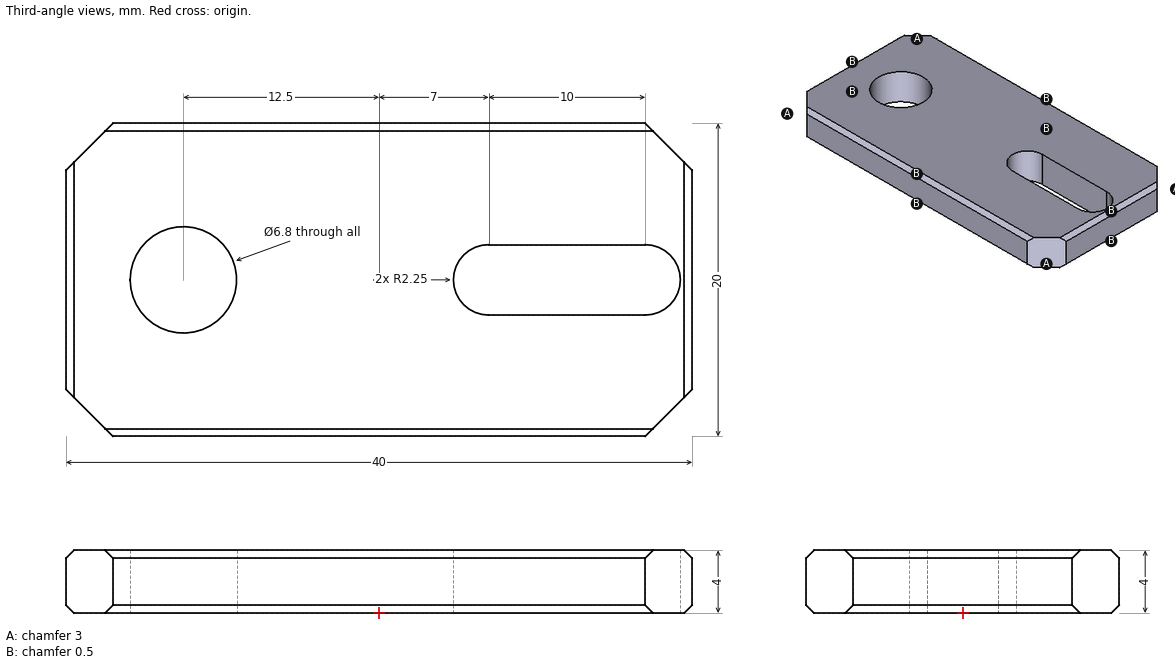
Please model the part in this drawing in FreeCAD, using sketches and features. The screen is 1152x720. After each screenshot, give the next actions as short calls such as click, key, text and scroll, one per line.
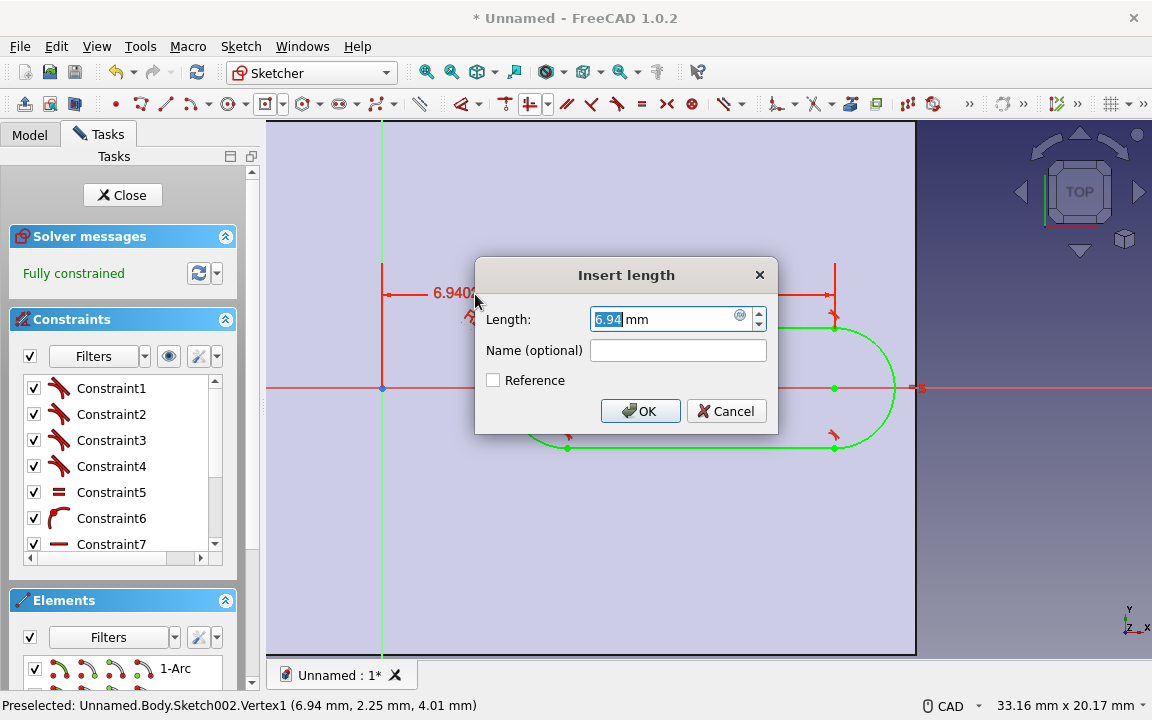
text(7)
key(Return)
key(Escape)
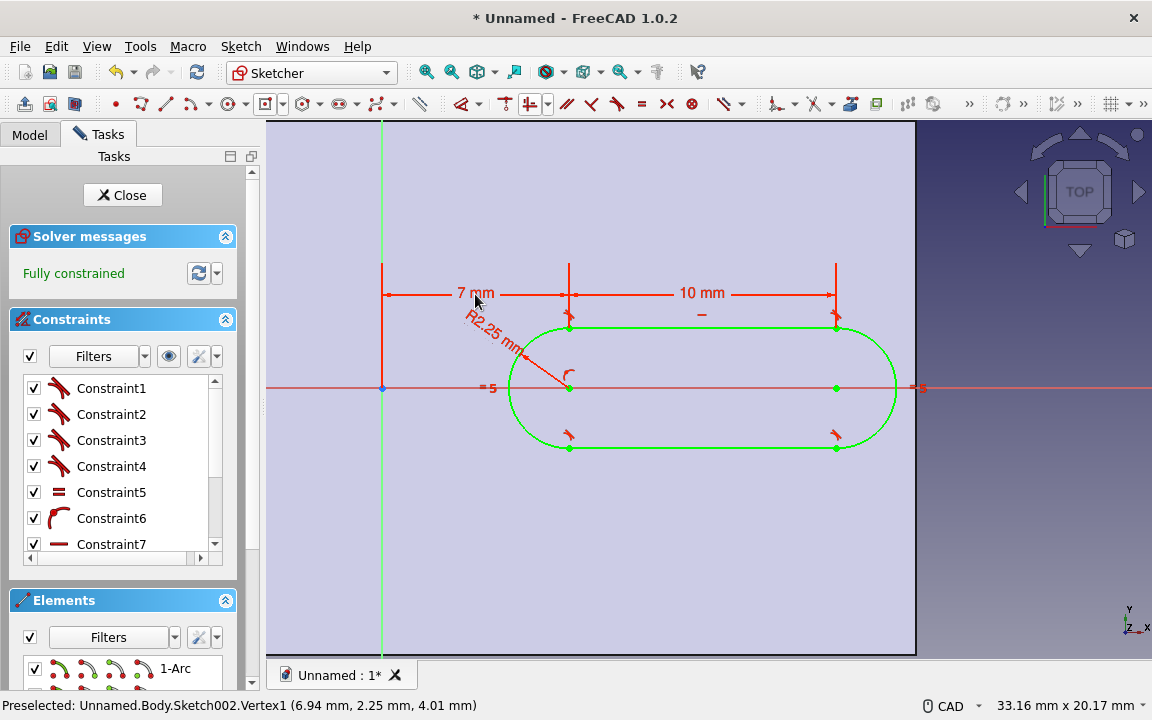
click(123, 195)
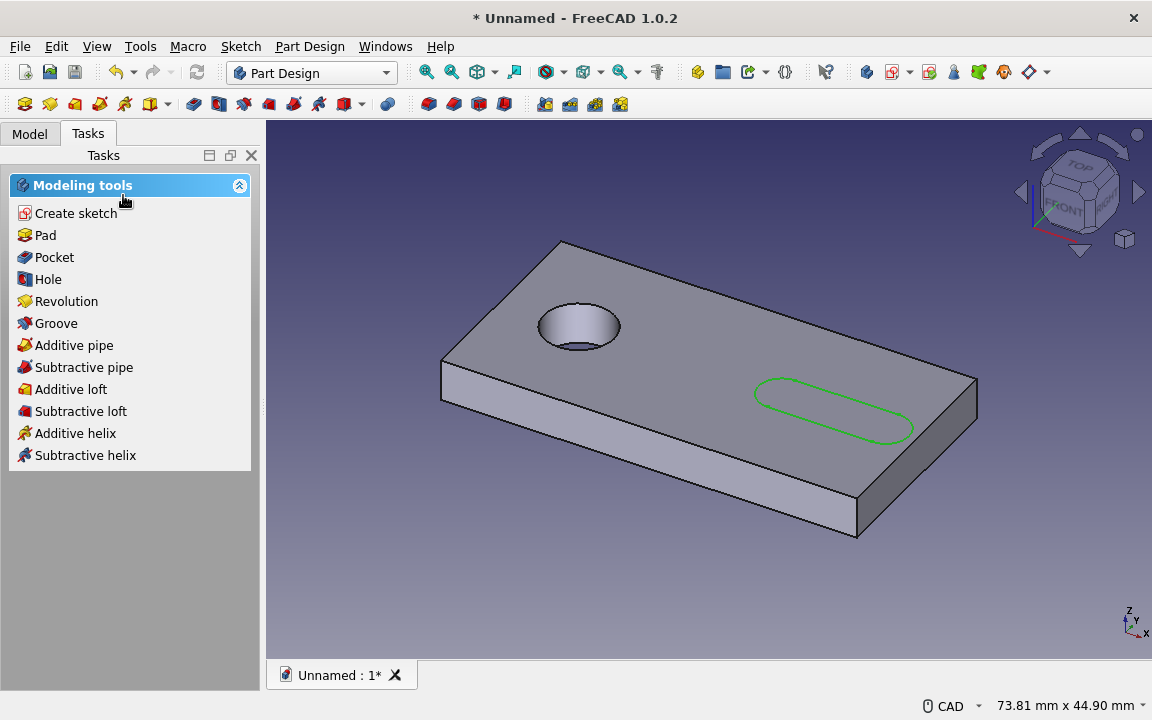
click(194, 104)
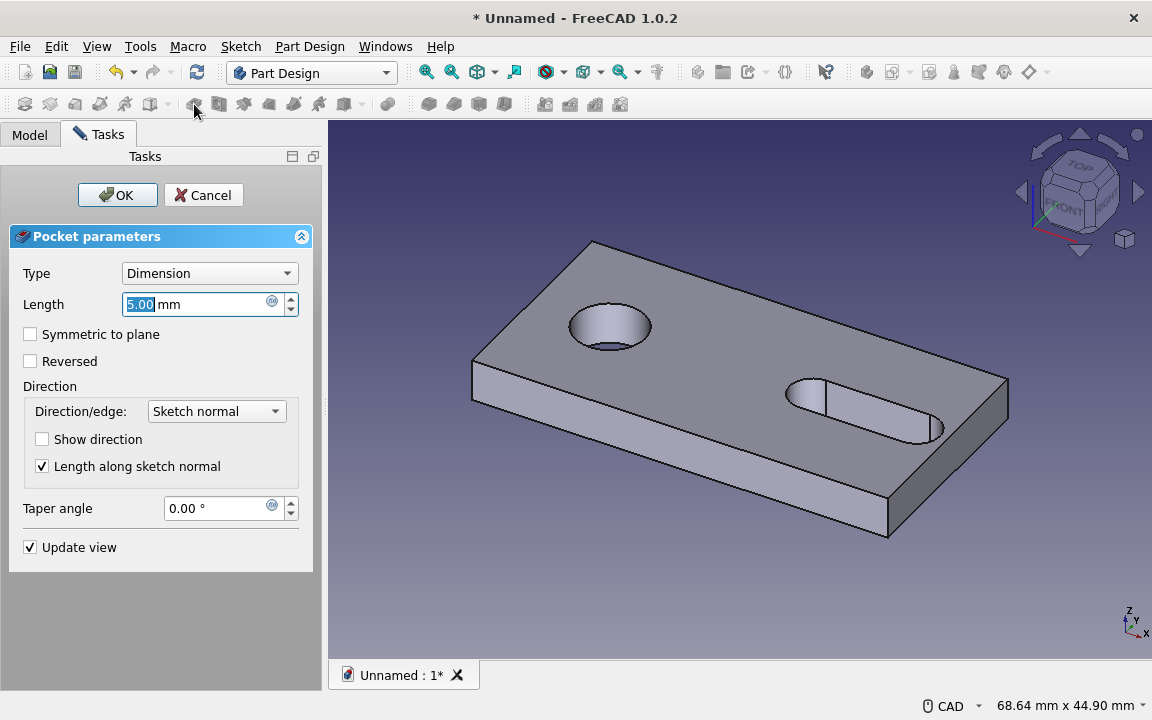
text(4)
key(Tab)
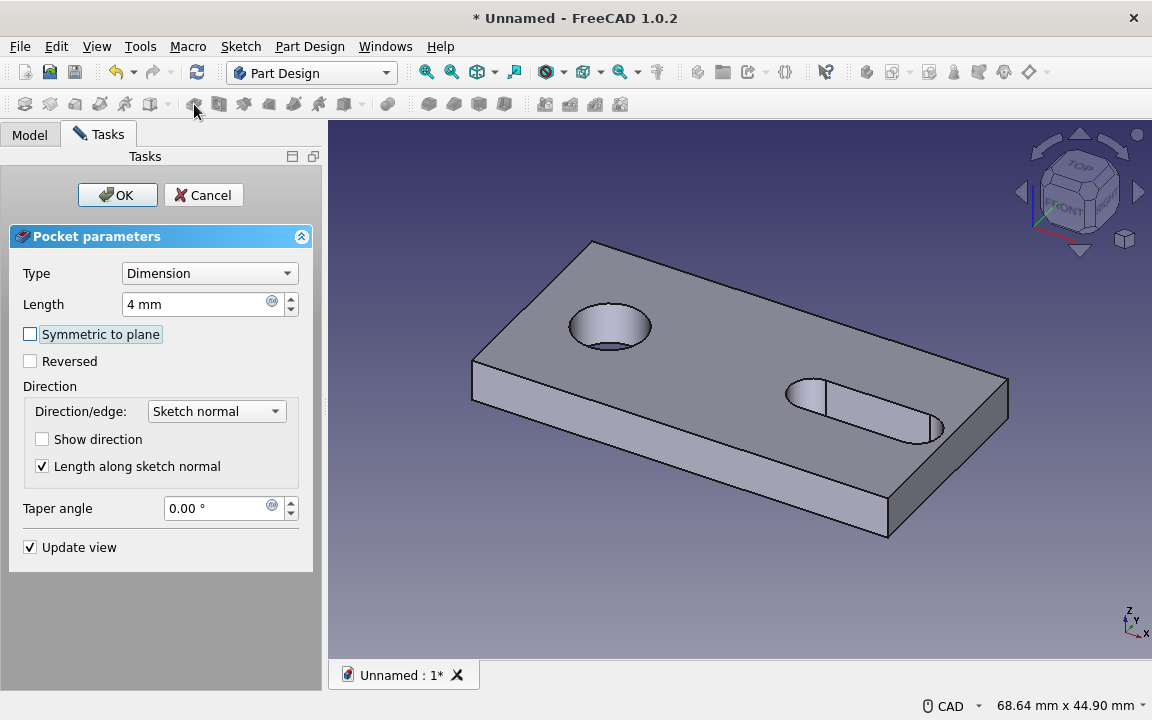
click(118, 195)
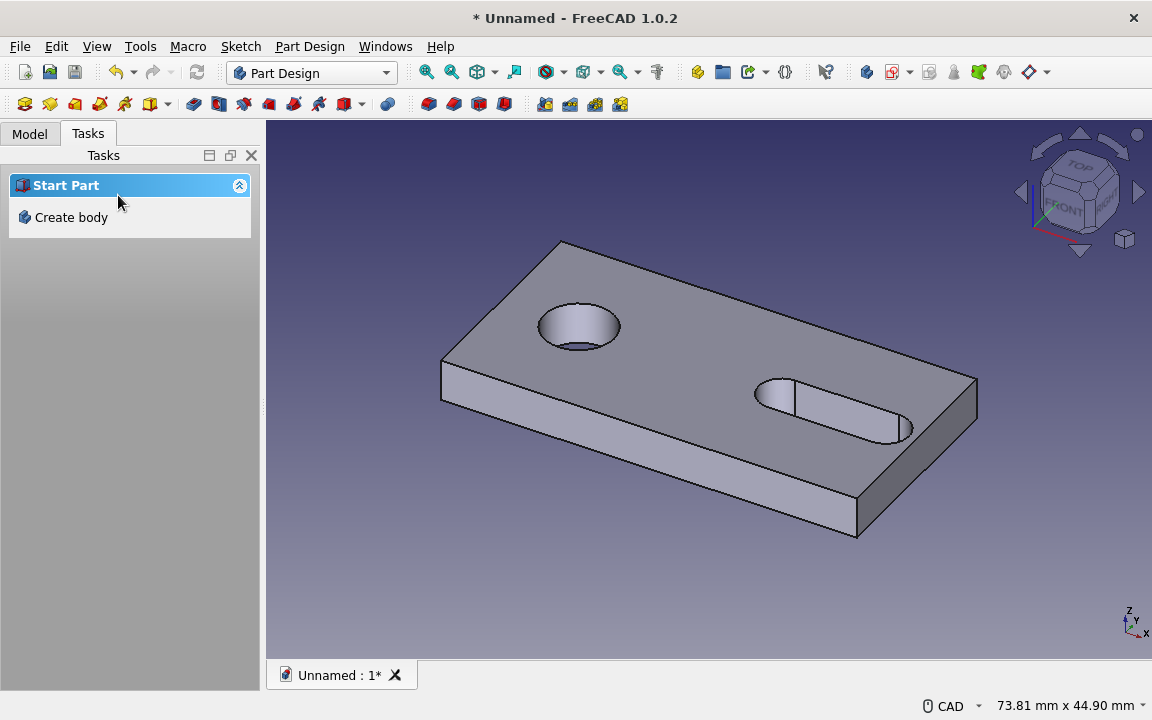
click(857, 517)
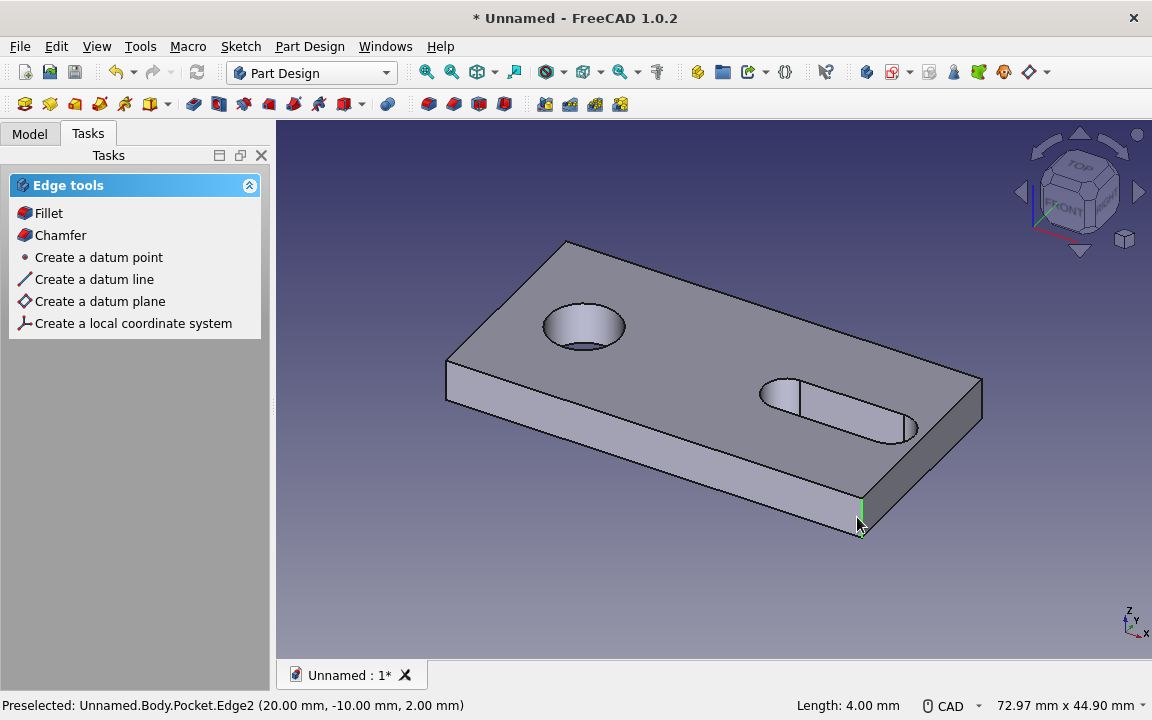
key(0)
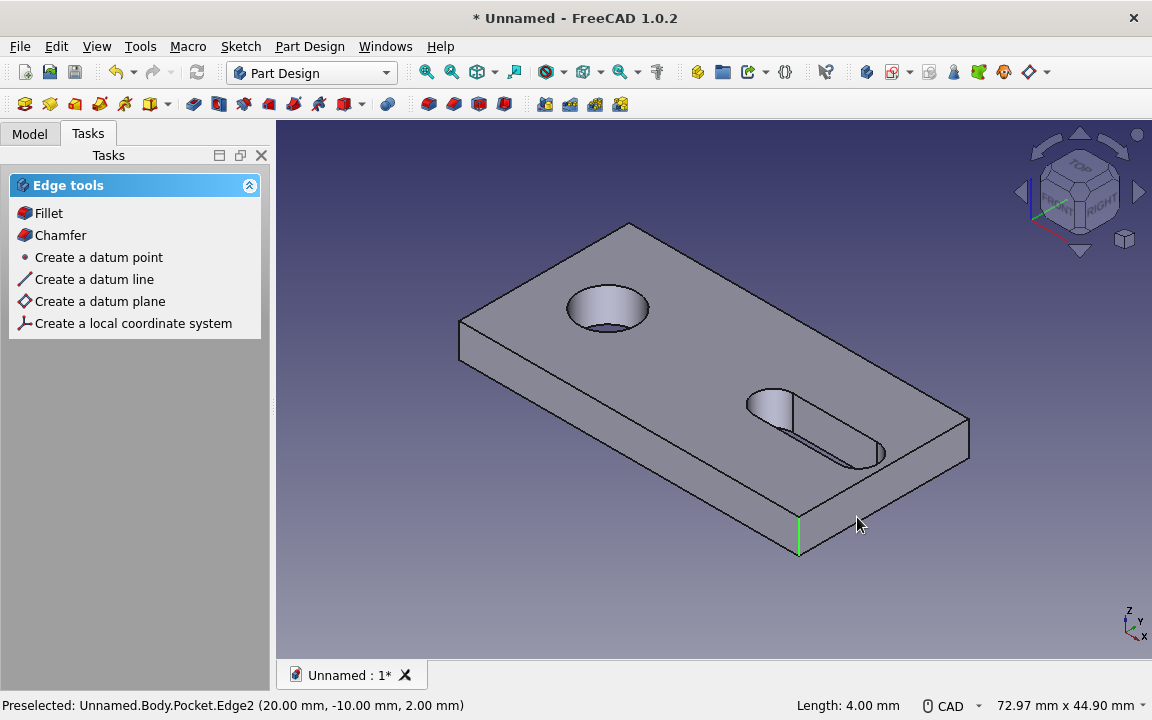
key(2)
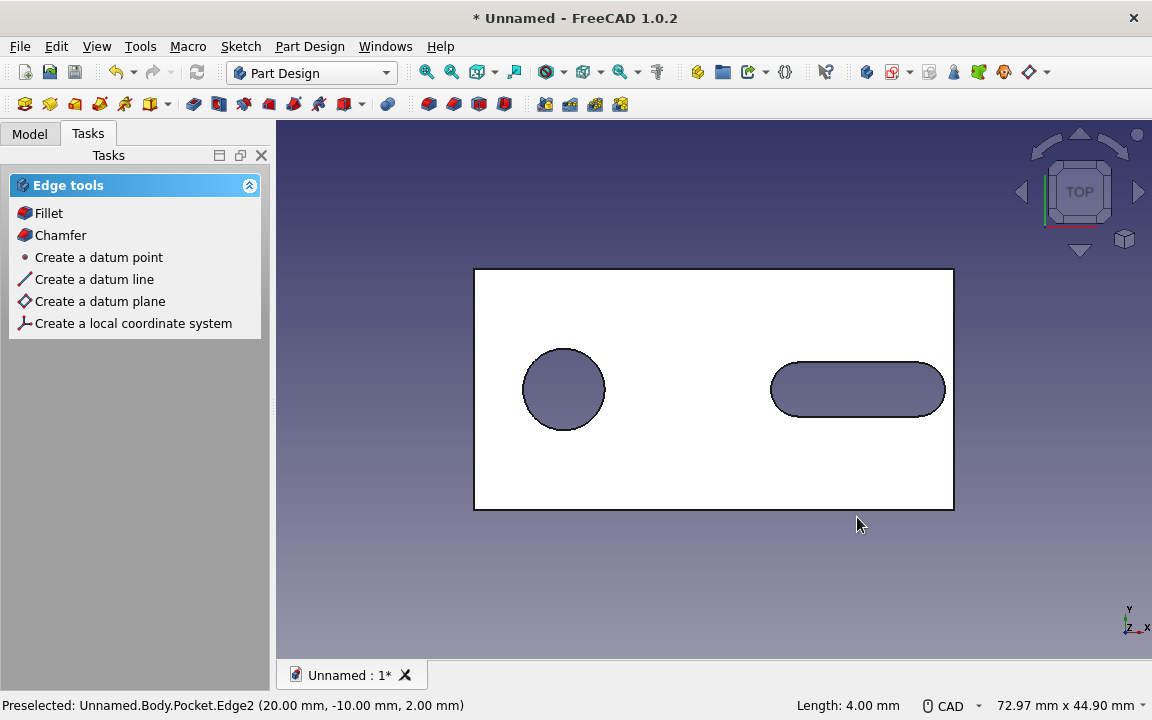
key(1)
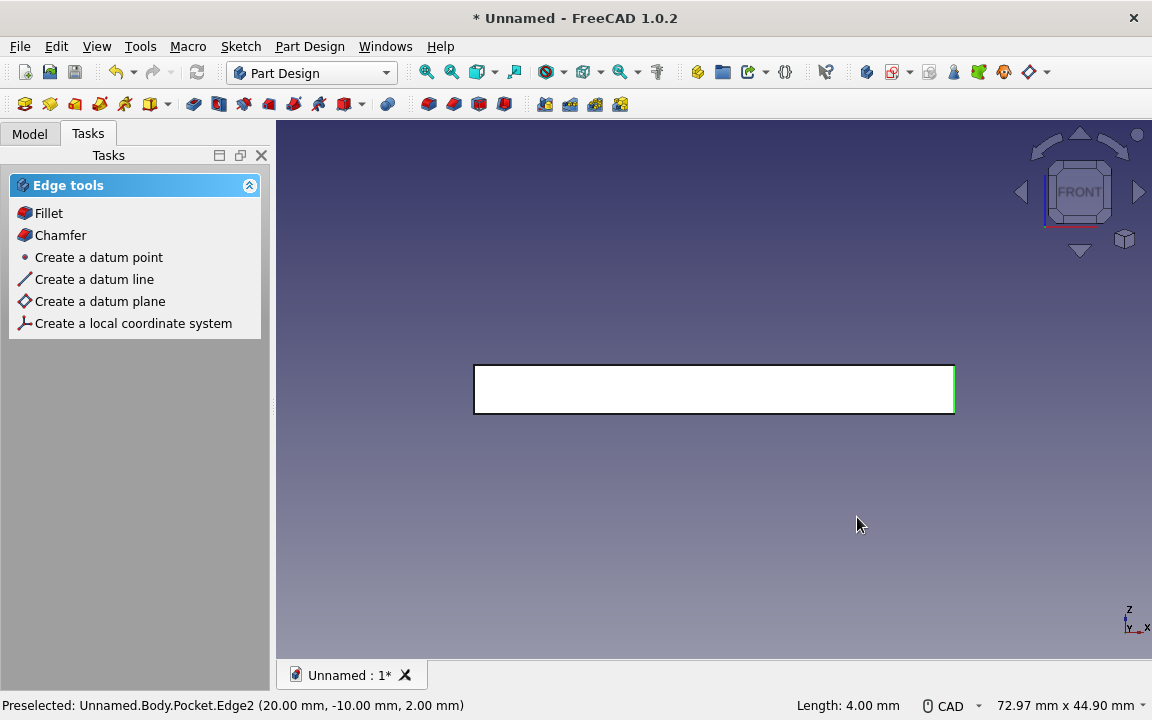
click(474, 388, ctrl)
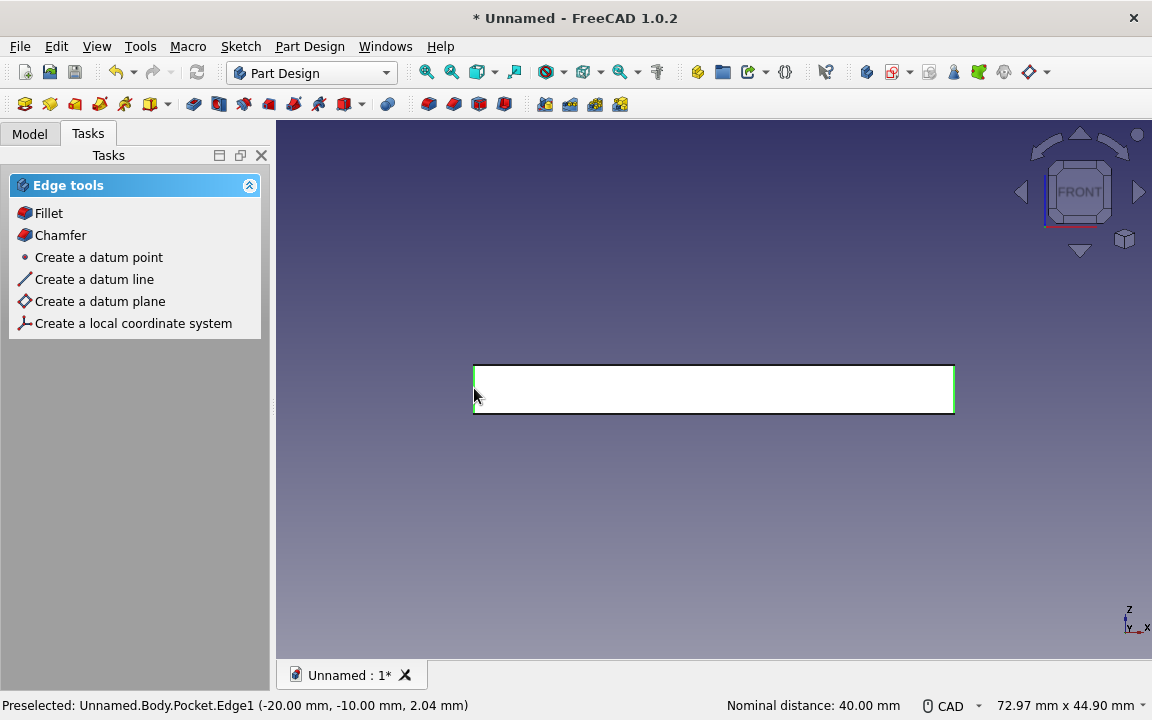
key(3)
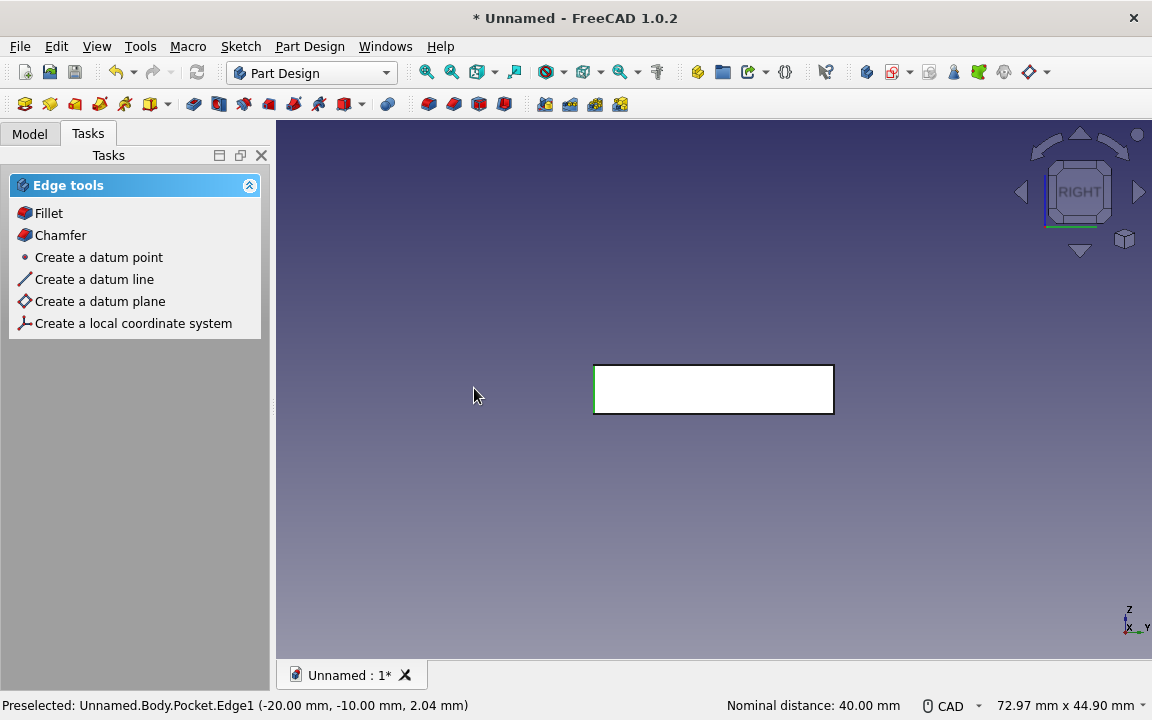
click(427, 72)